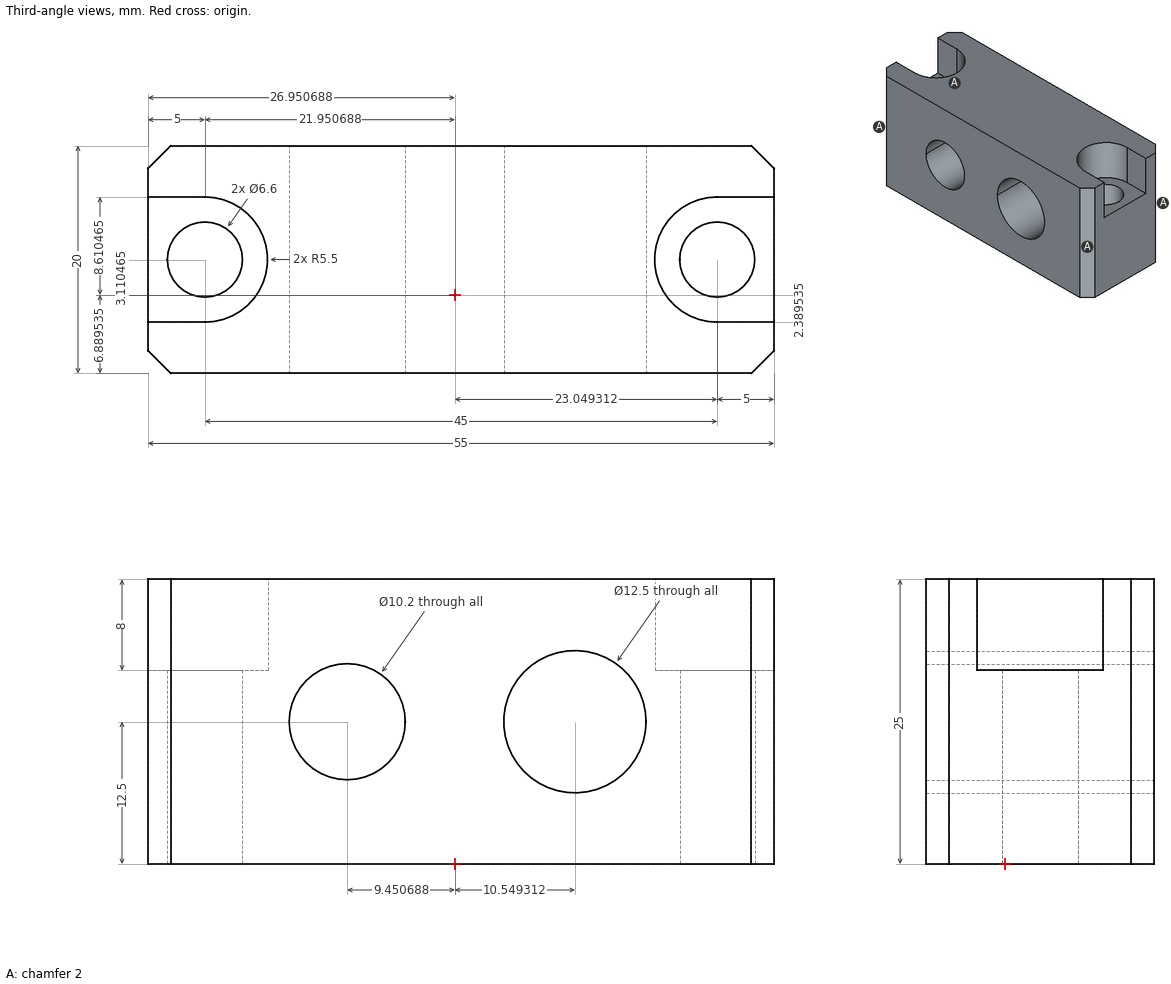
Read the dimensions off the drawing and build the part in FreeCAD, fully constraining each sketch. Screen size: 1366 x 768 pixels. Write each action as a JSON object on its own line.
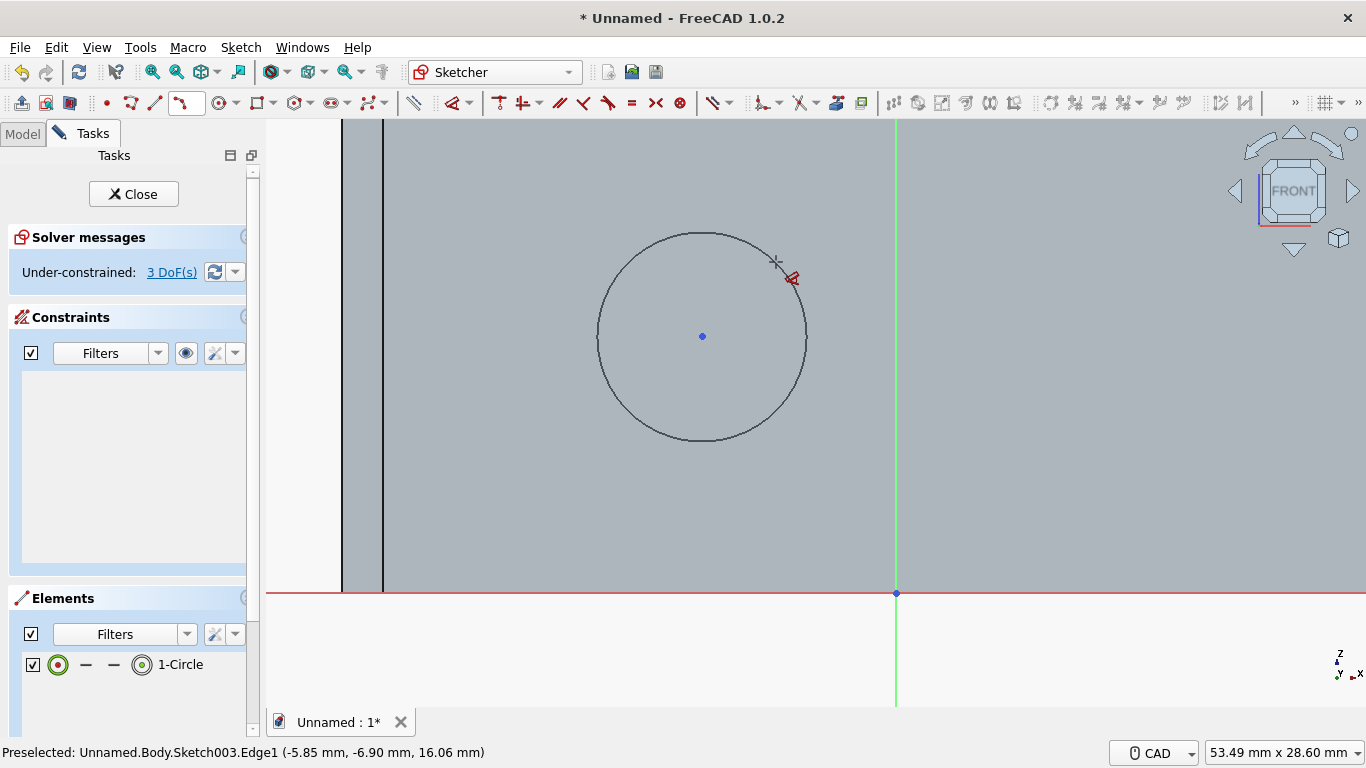
{"action": "left_click", "coordinate": [776, 263]}
{"action": "left_click", "coordinate": [799, 240]}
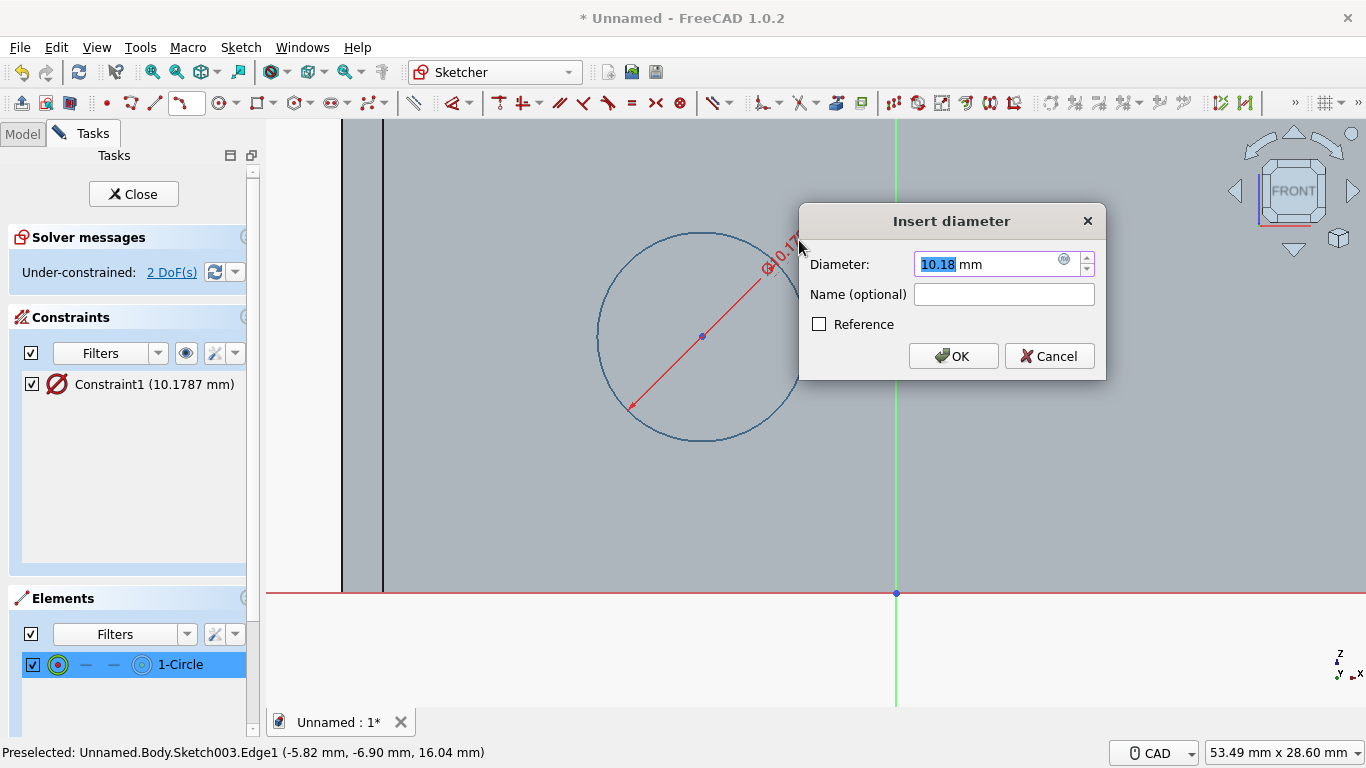
{"action": "type", "text": "10.2"}
{"action": "key", "text": "Return"}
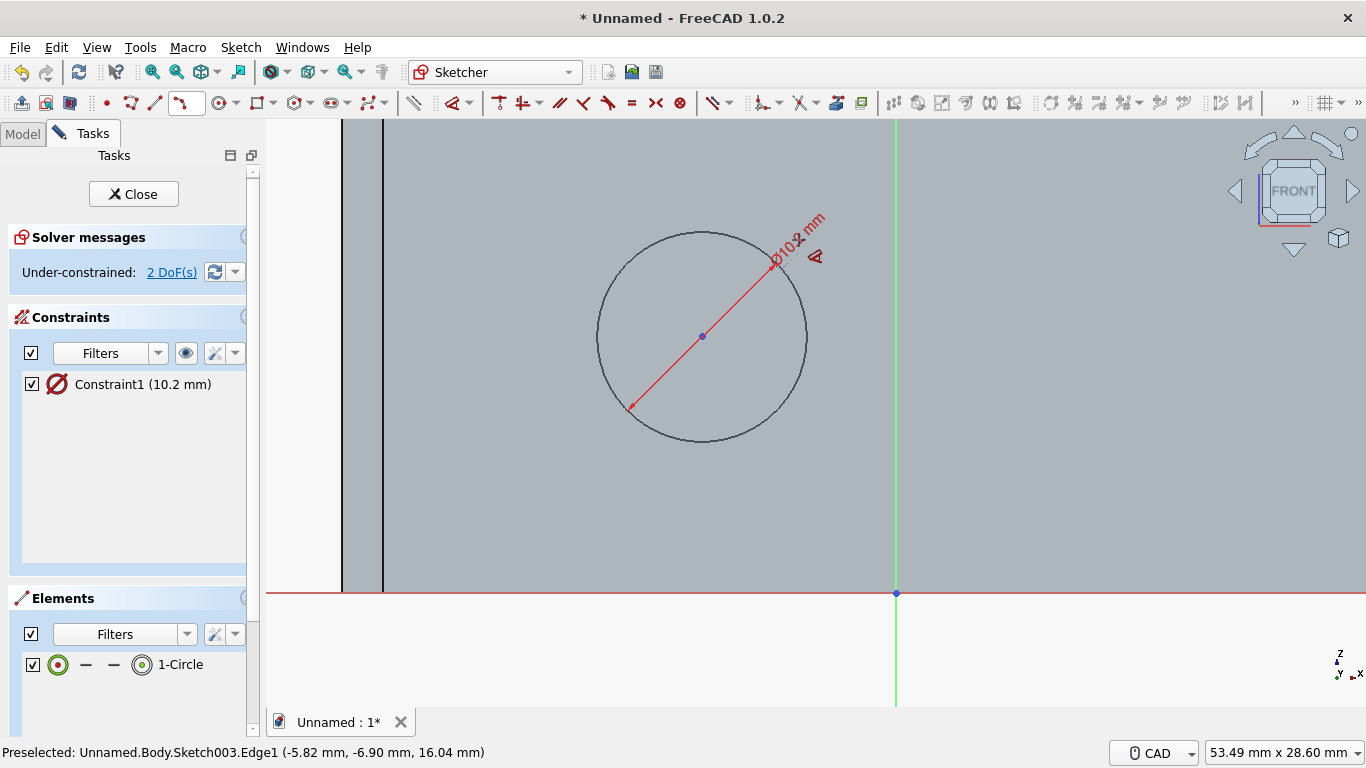
{"action": "left_click", "coordinate": [702, 337]}
{"action": "left_click", "coordinate": [930, 465]}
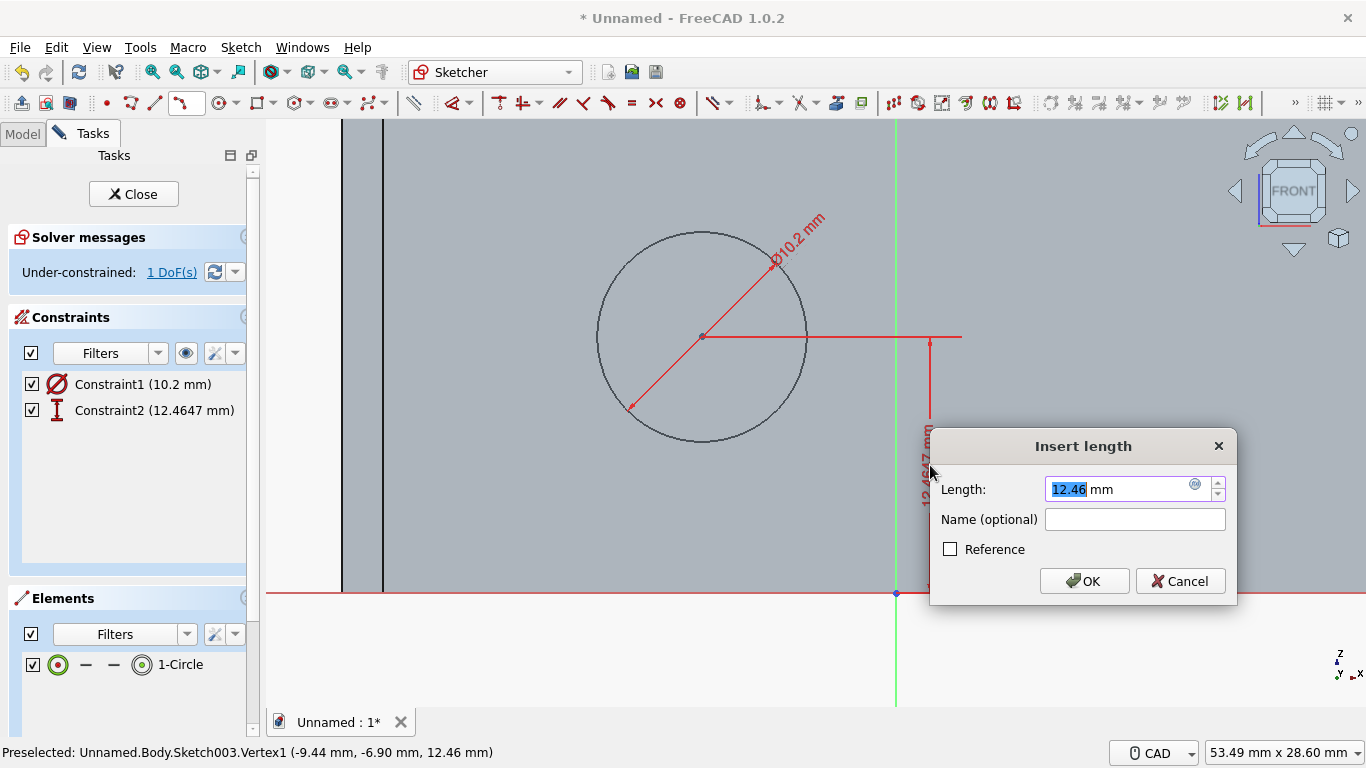
{"action": "type", "text": "12.5"}
{"action": "key", "text": "Return"}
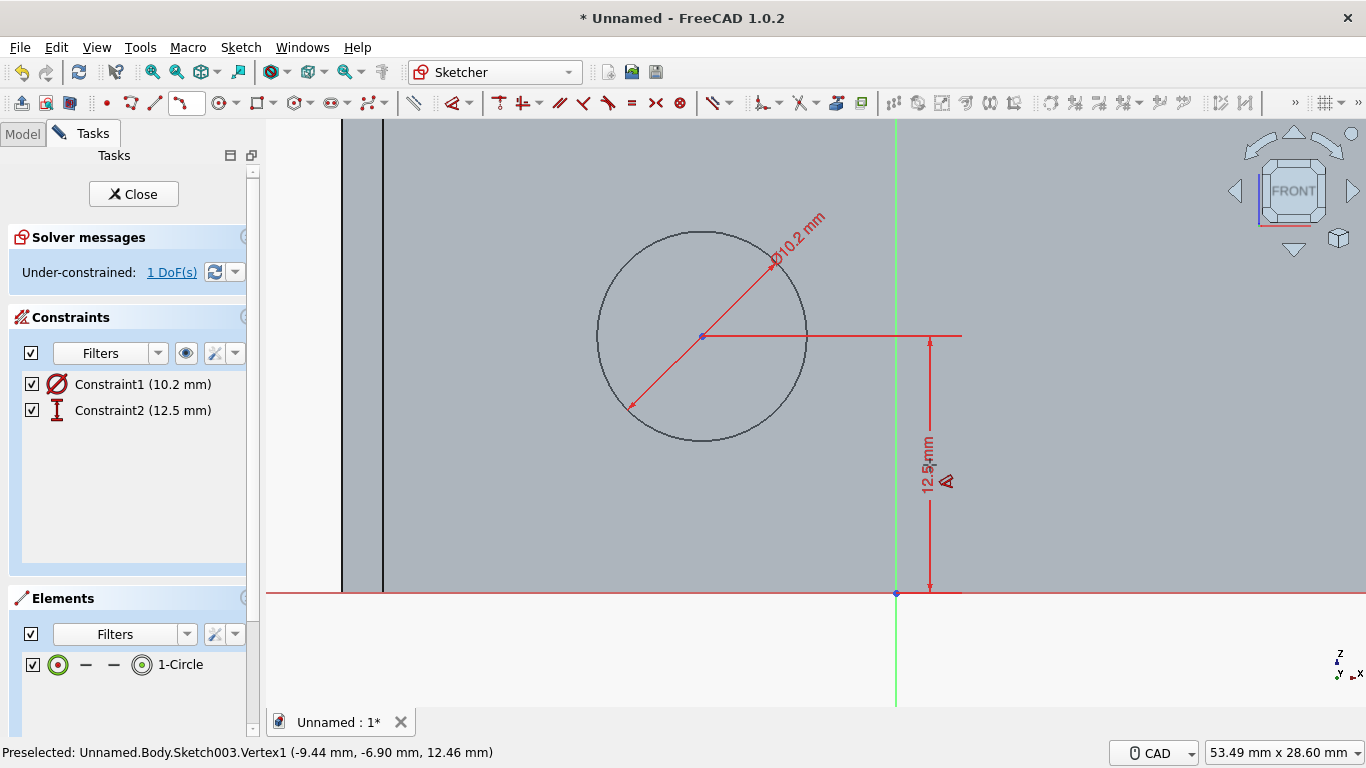
{"action": "left_click", "coordinate": [702, 336]}
{"action": "left_click", "coordinate": [799, 627]}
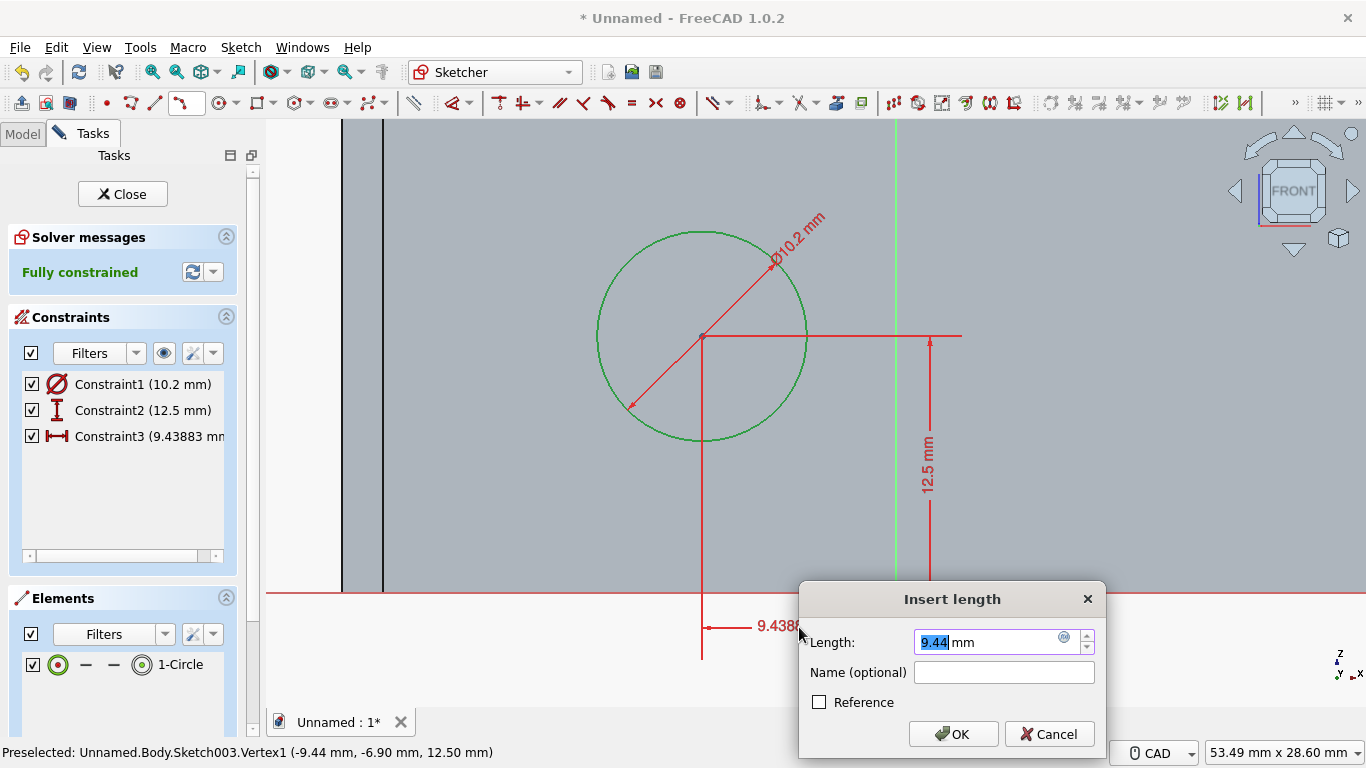
{"action": "type", "text": "9.450688"}
{"action": "key", "text": "Return"}
{"action": "key", "text": "Escape"}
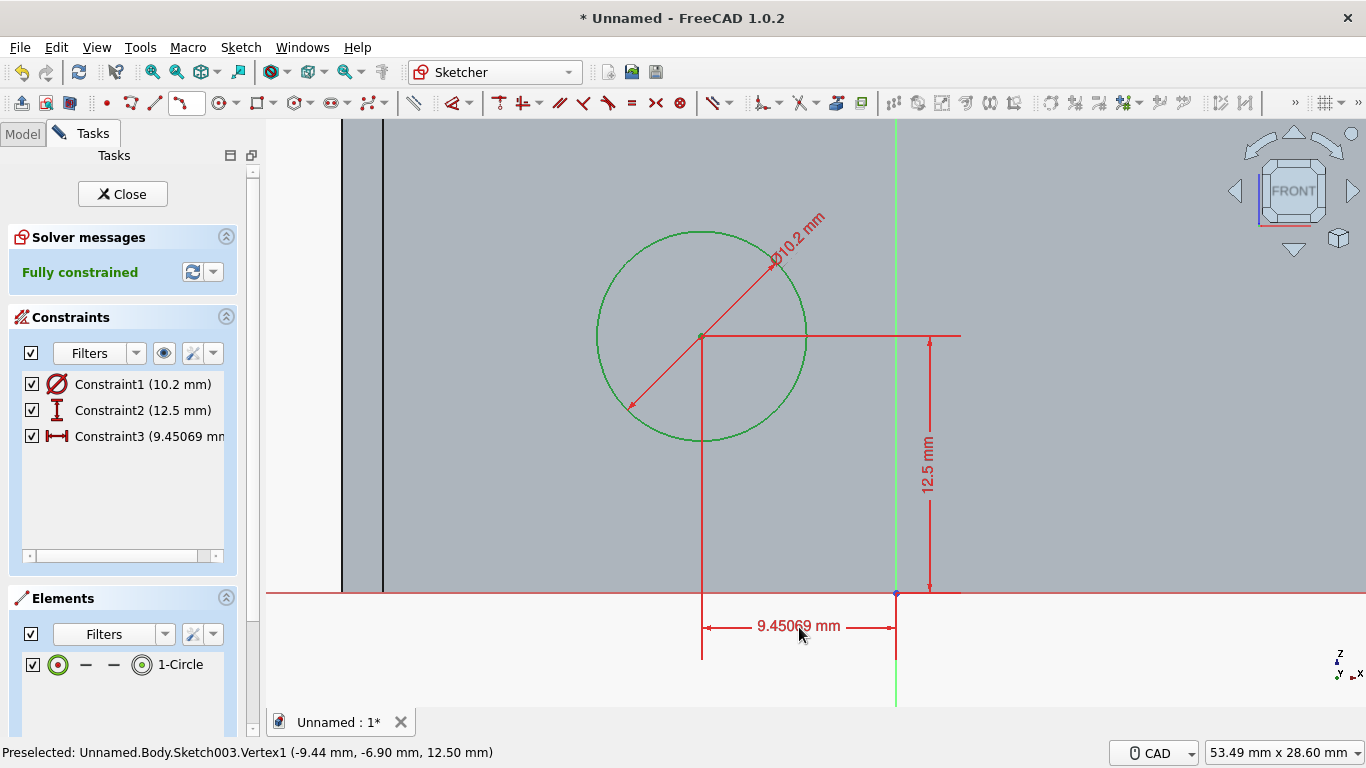
{"action": "left_click", "coordinate": [123, 194]}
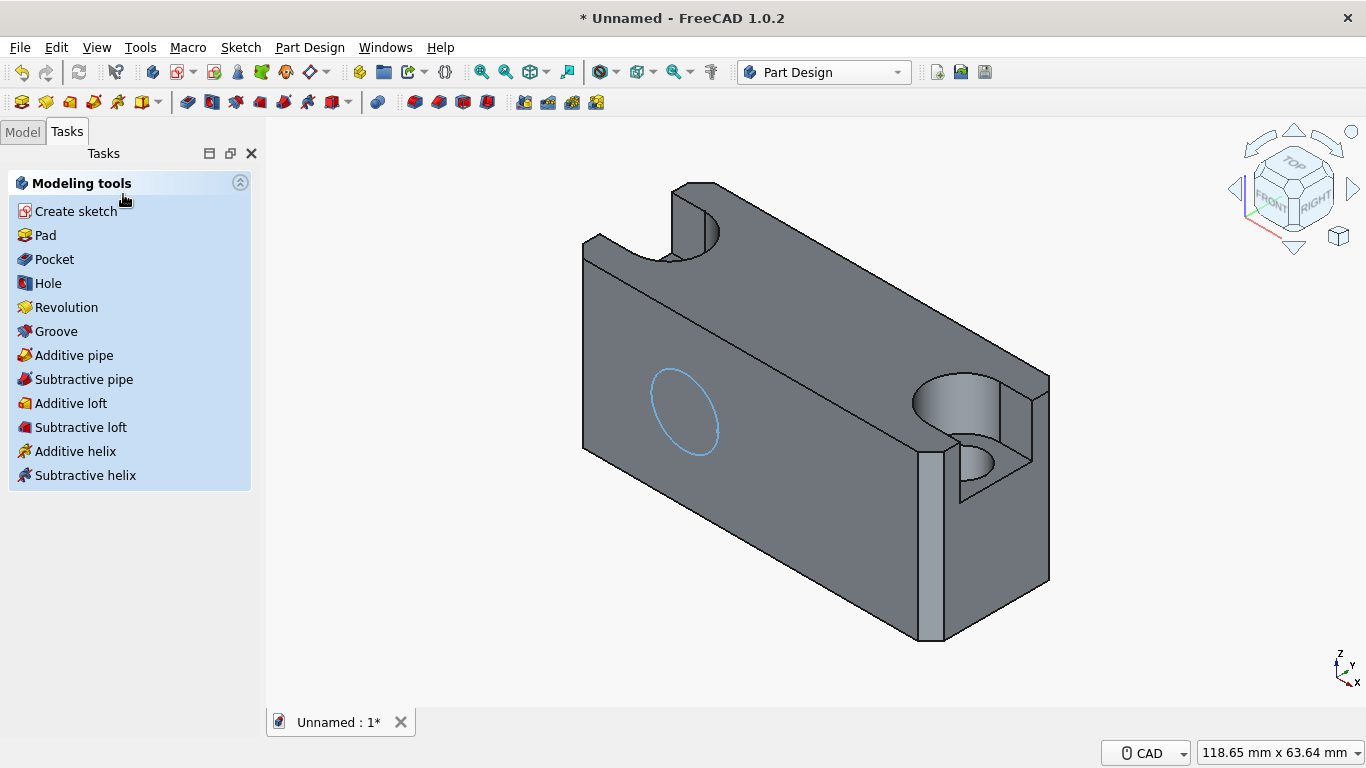
{"action": "left_click", "coordinate": [212, 102]}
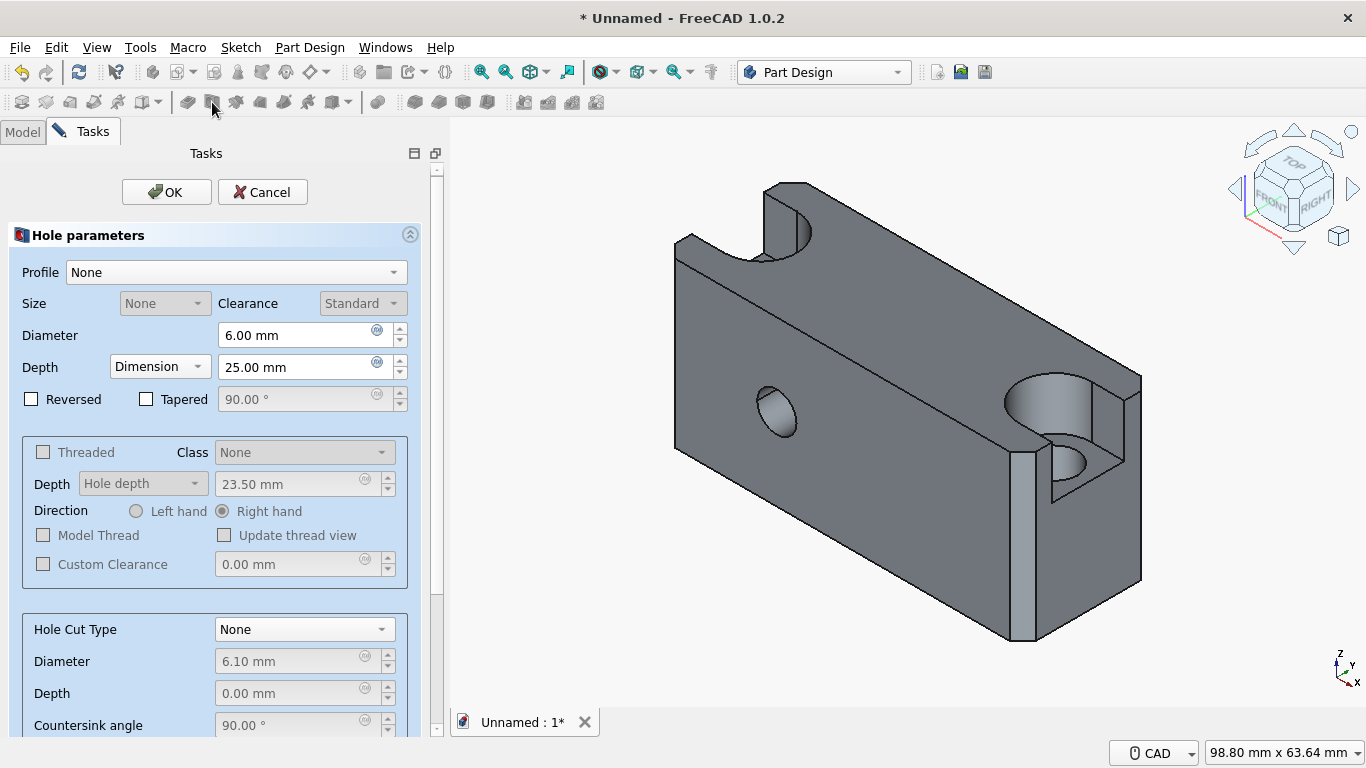
{"action": "triple_click", "coordinate": [305, 335]}